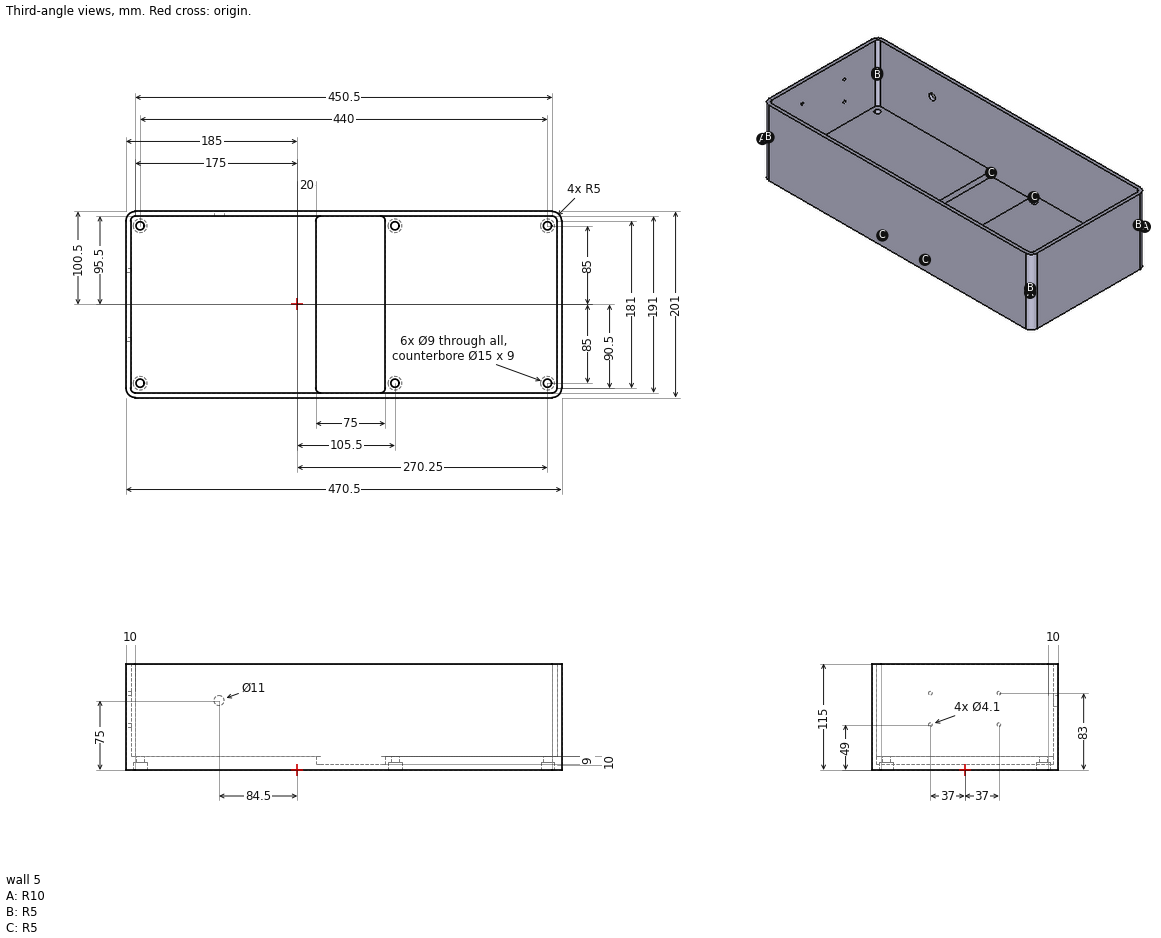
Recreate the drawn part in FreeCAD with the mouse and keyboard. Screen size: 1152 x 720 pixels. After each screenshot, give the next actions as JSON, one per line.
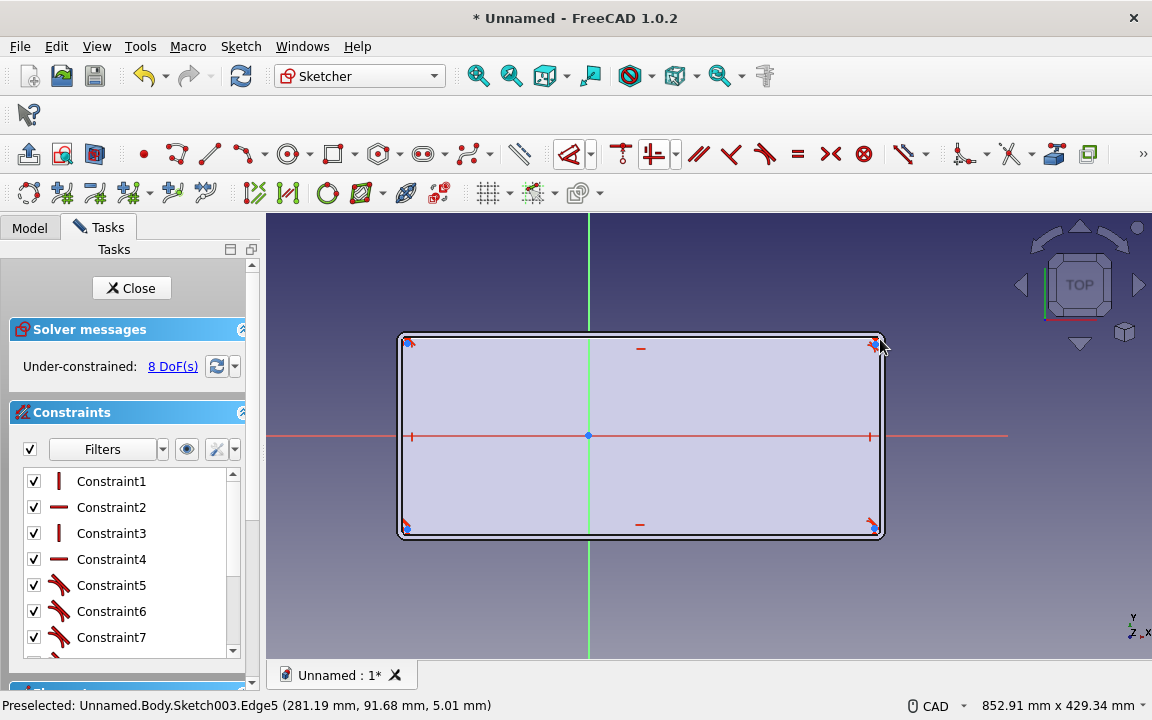
{"action": "scroll", "coordinate": [404, 338], "scroll_direction": "up", "scroll_amount": 9}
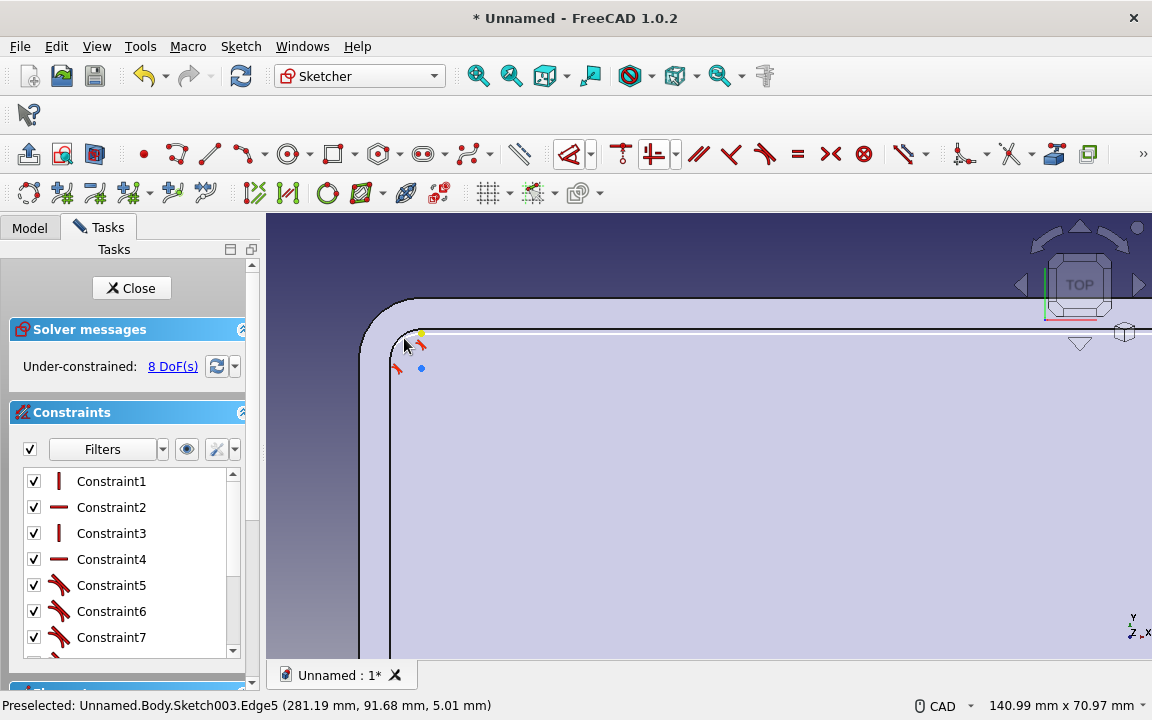
{"action": "left_click", "coordinate": [406, 338]}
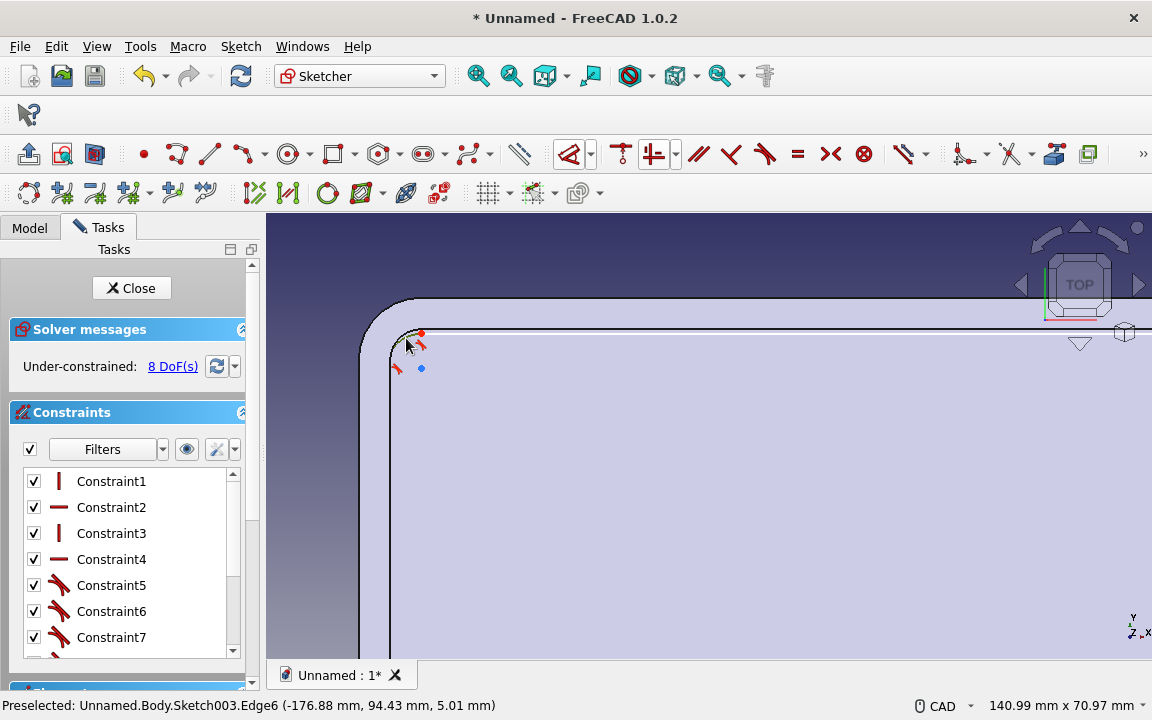
{"action": "scroll", "coordinate": [404, 338], "scroll_direction": "down", "scroll_amount": 9}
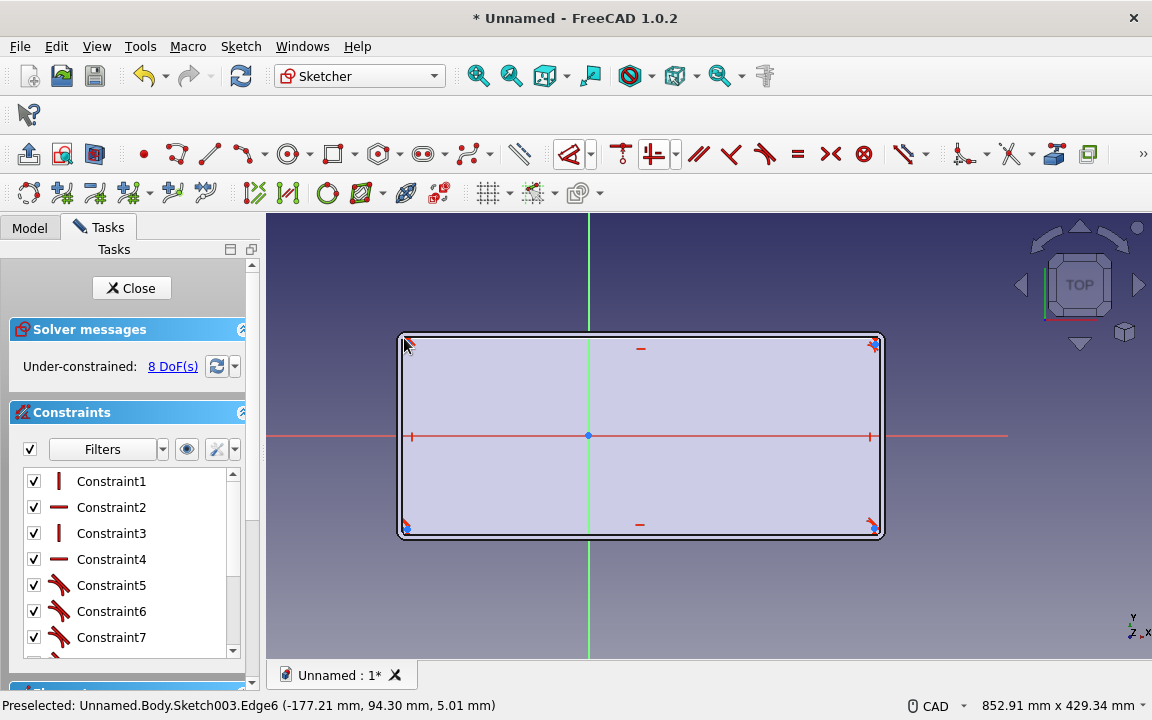
{"action": "scroll", "coordinate": [402, 533], "scroll_direction": "up", "scroll_amount": 9}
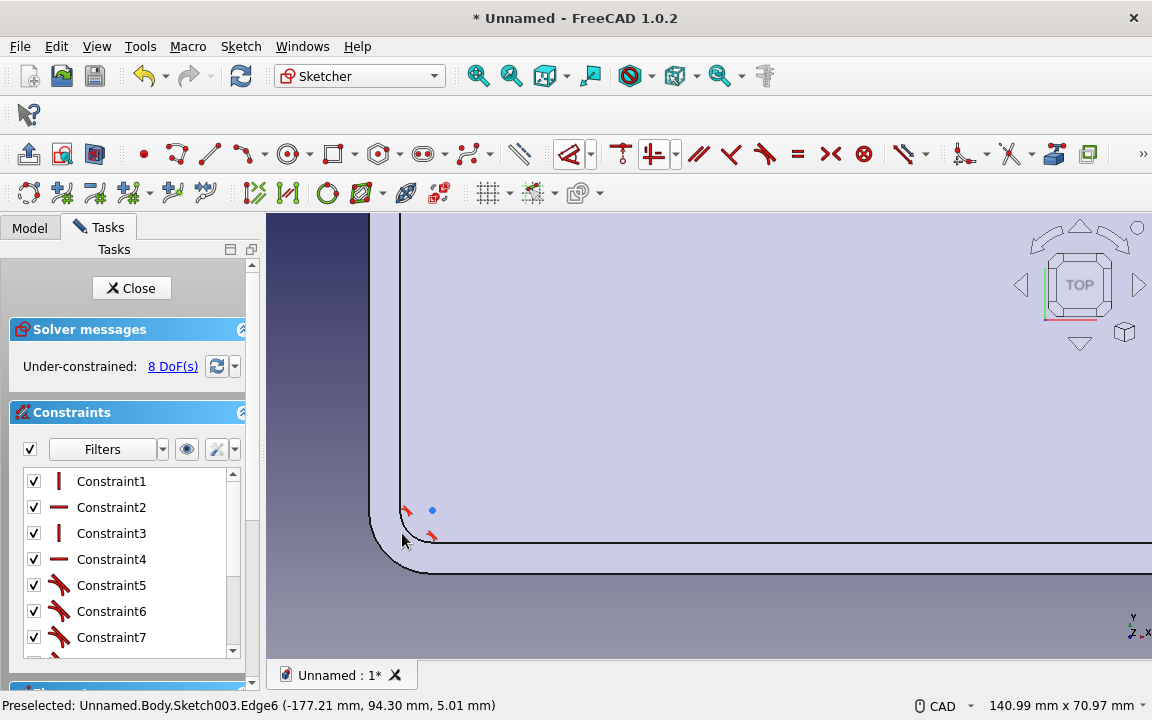
{"action": "left_click", "coordinate": [400, 527]}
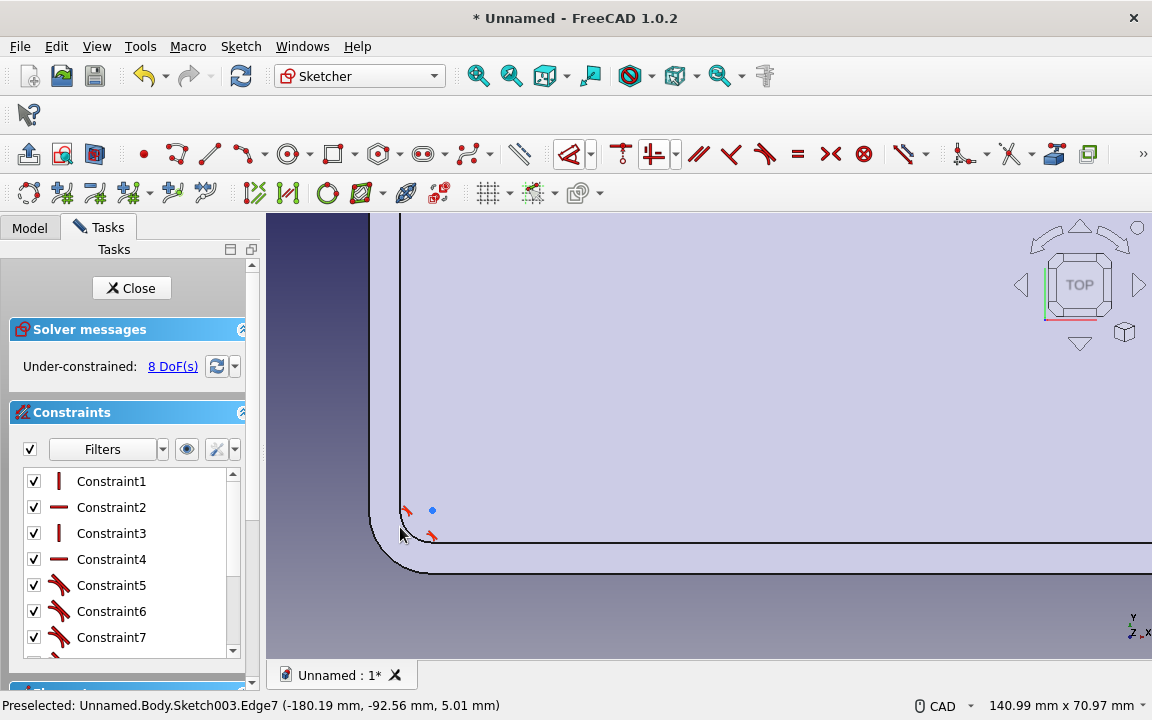
{"action": "scroll", "coordinate": [402, 534], "scroll_direction": "down", "scroll_amount": 9}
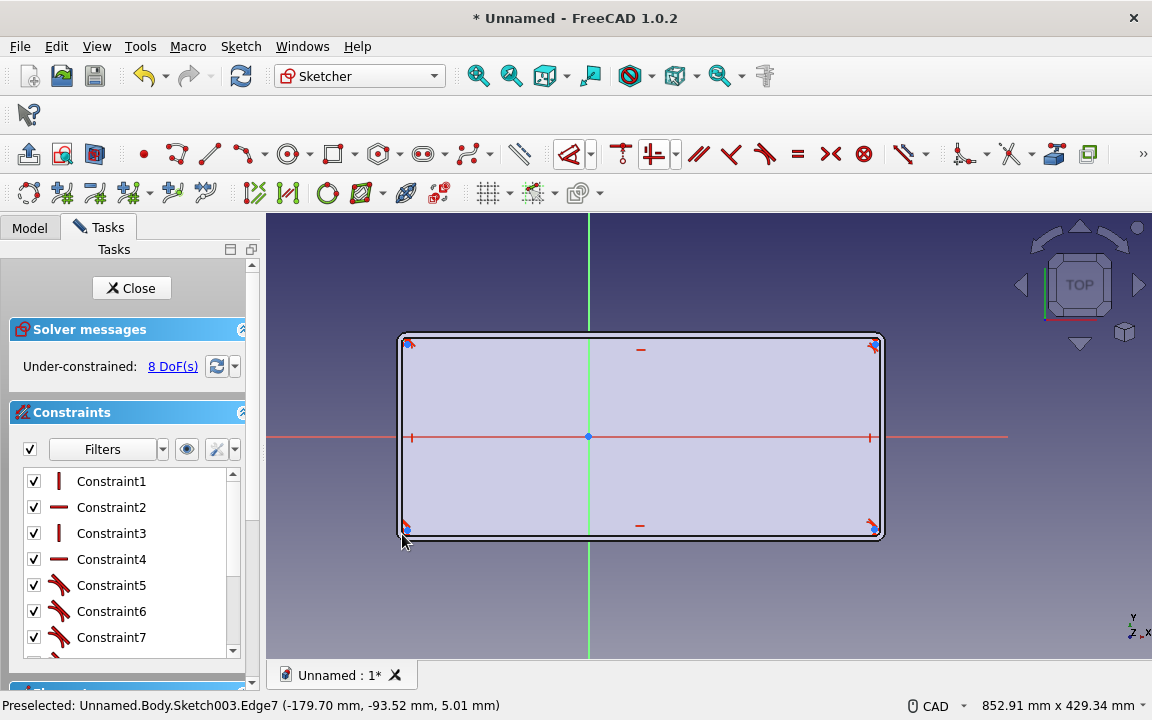
{"action": "scroll", "coordinate": [878, 536], "scroll_direction": "up", "scroll_amount": 7}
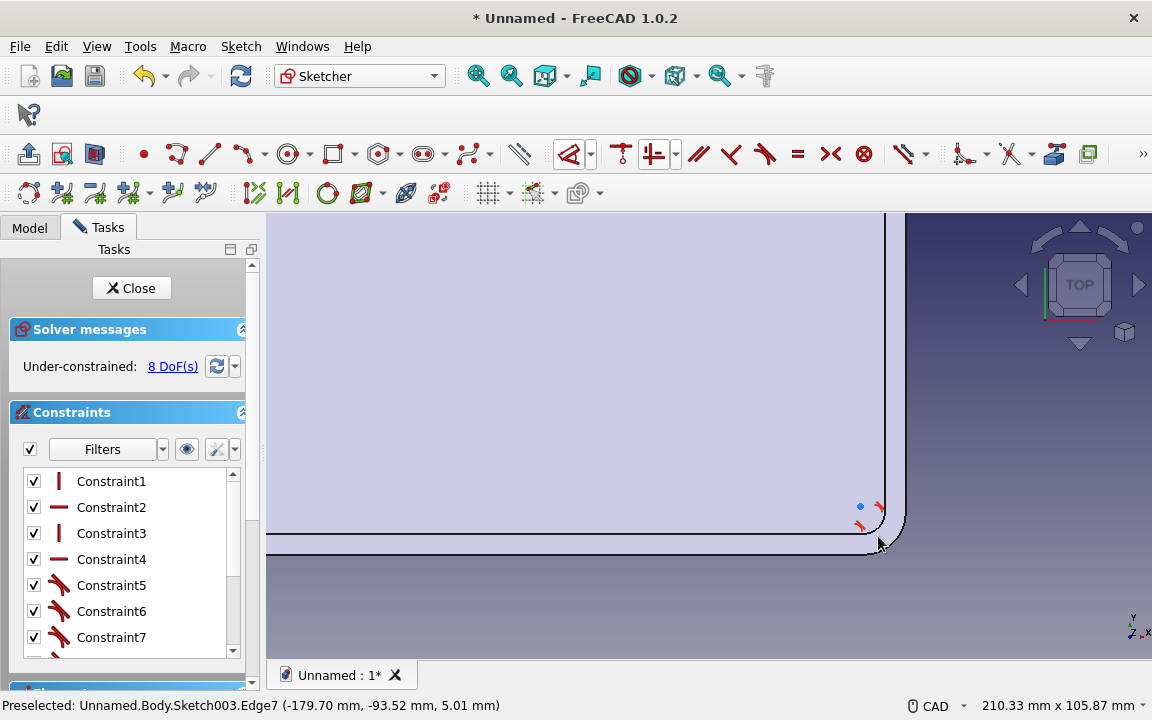
{"action": "left_click", "coordinate": [875, 533]}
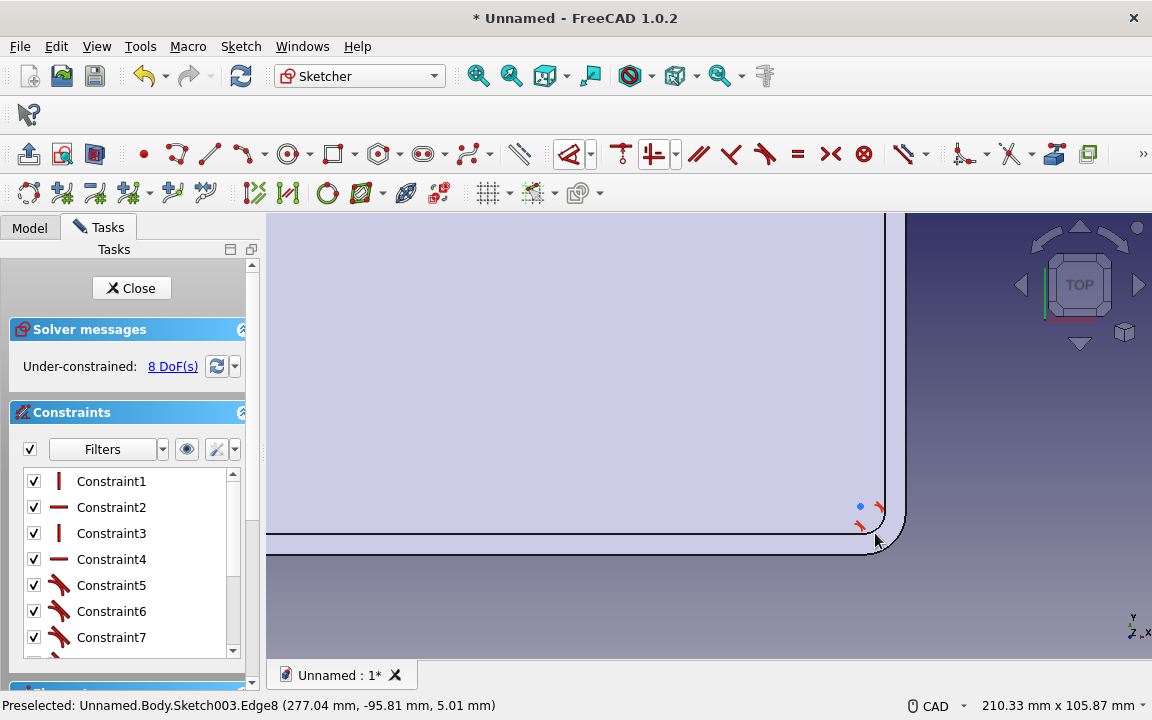
{"action": "key", "text": "e"}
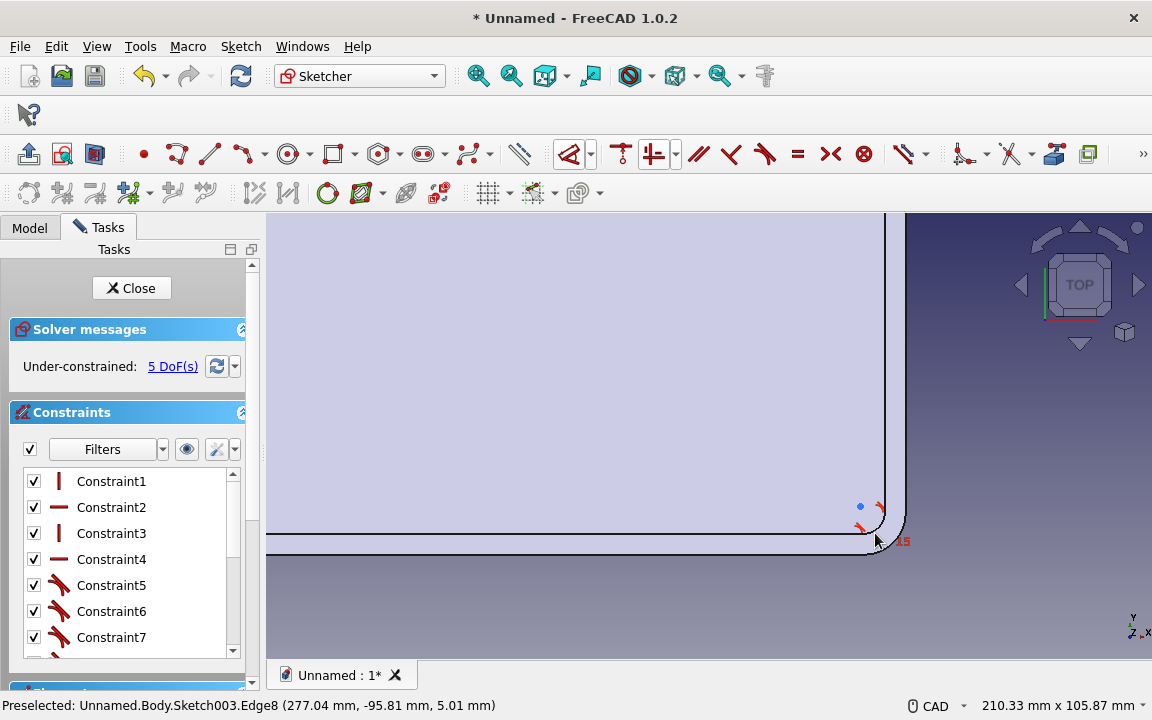
{"action": "key", "text": "d"}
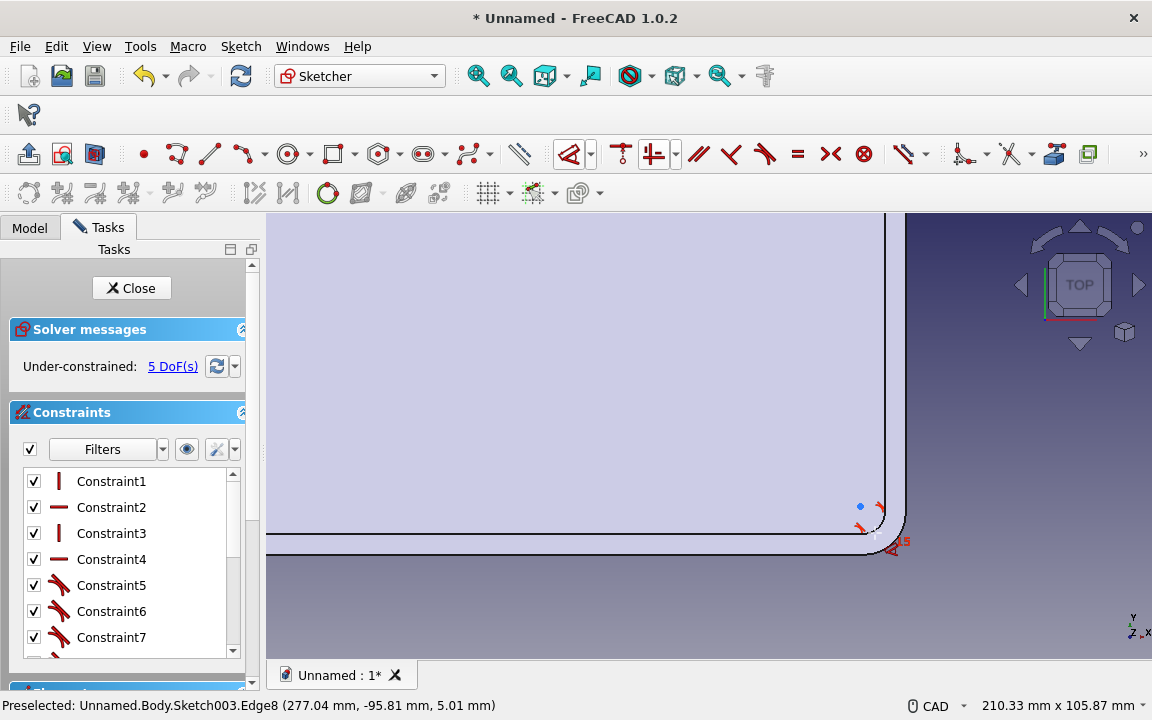
{"action": "scroll", "coordinate": [878, 536], "scroll_direction": "down", "scroll_amount": 7}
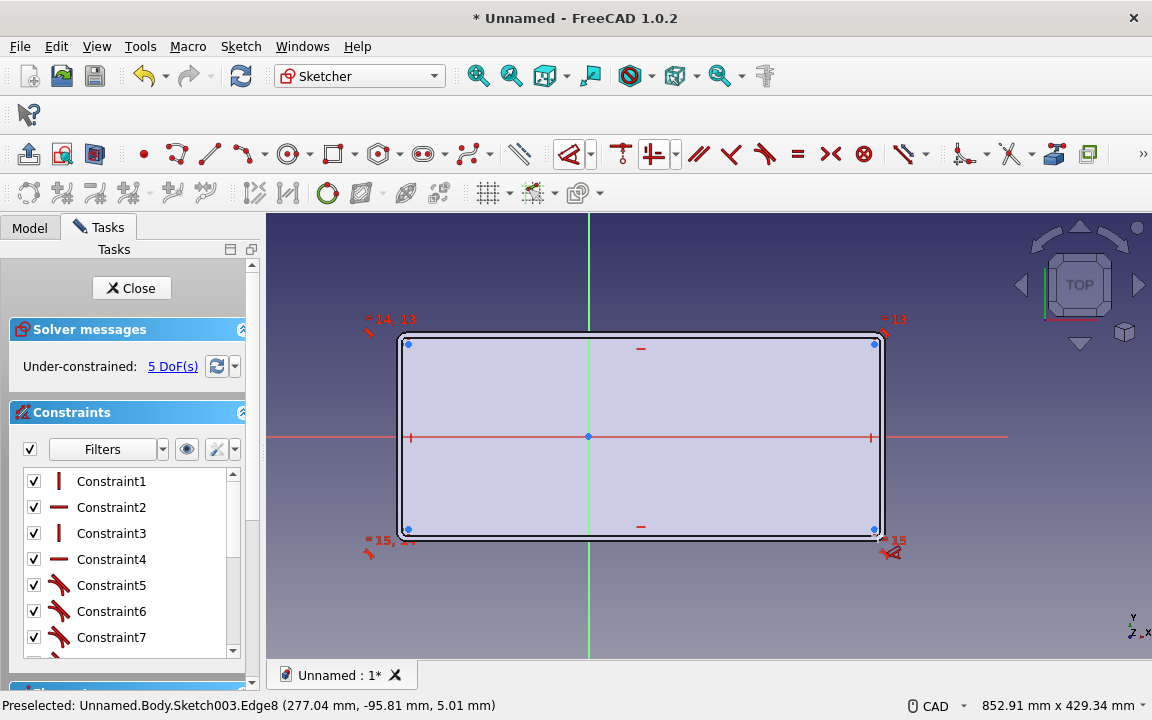
{"action": "scroll", "coordinate": [881, 341], "scroll_direction": "up", "scroll_amount": 11}